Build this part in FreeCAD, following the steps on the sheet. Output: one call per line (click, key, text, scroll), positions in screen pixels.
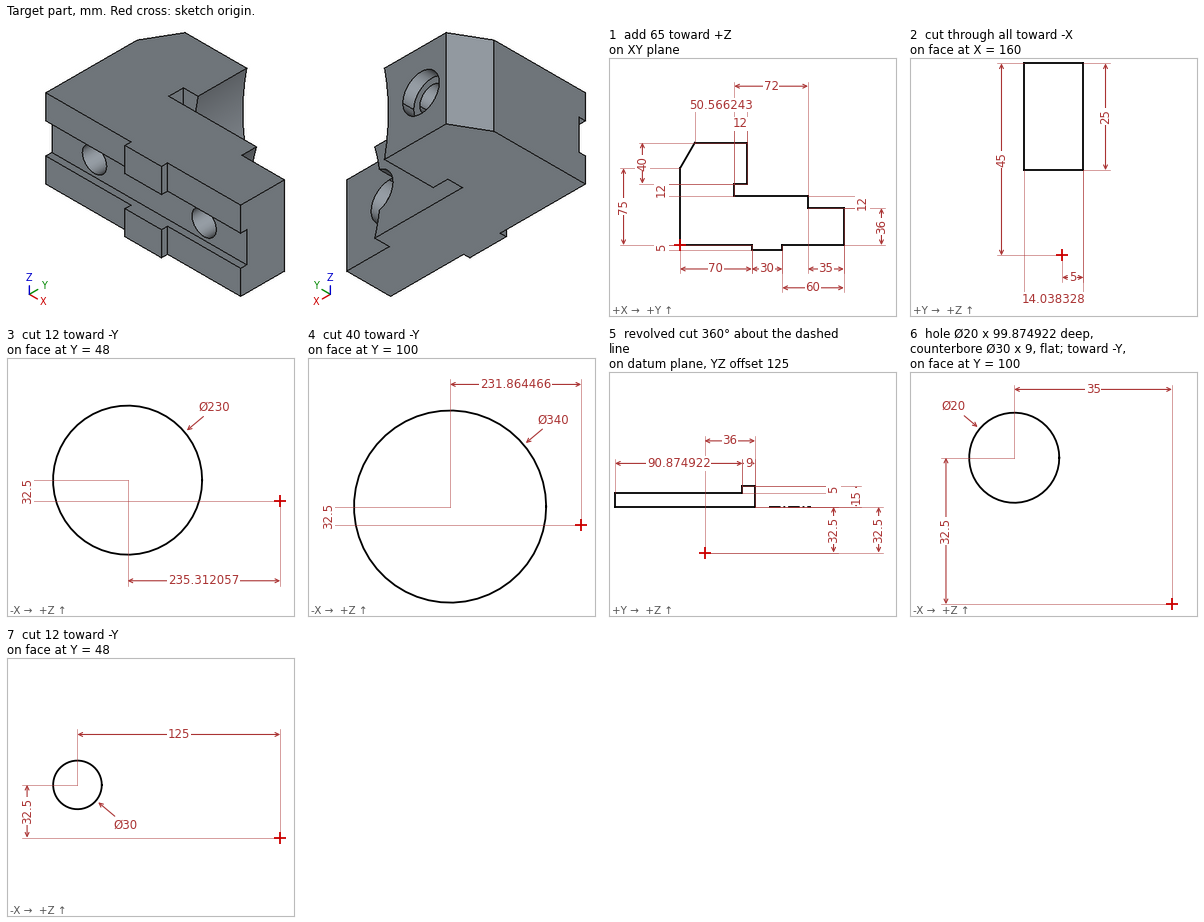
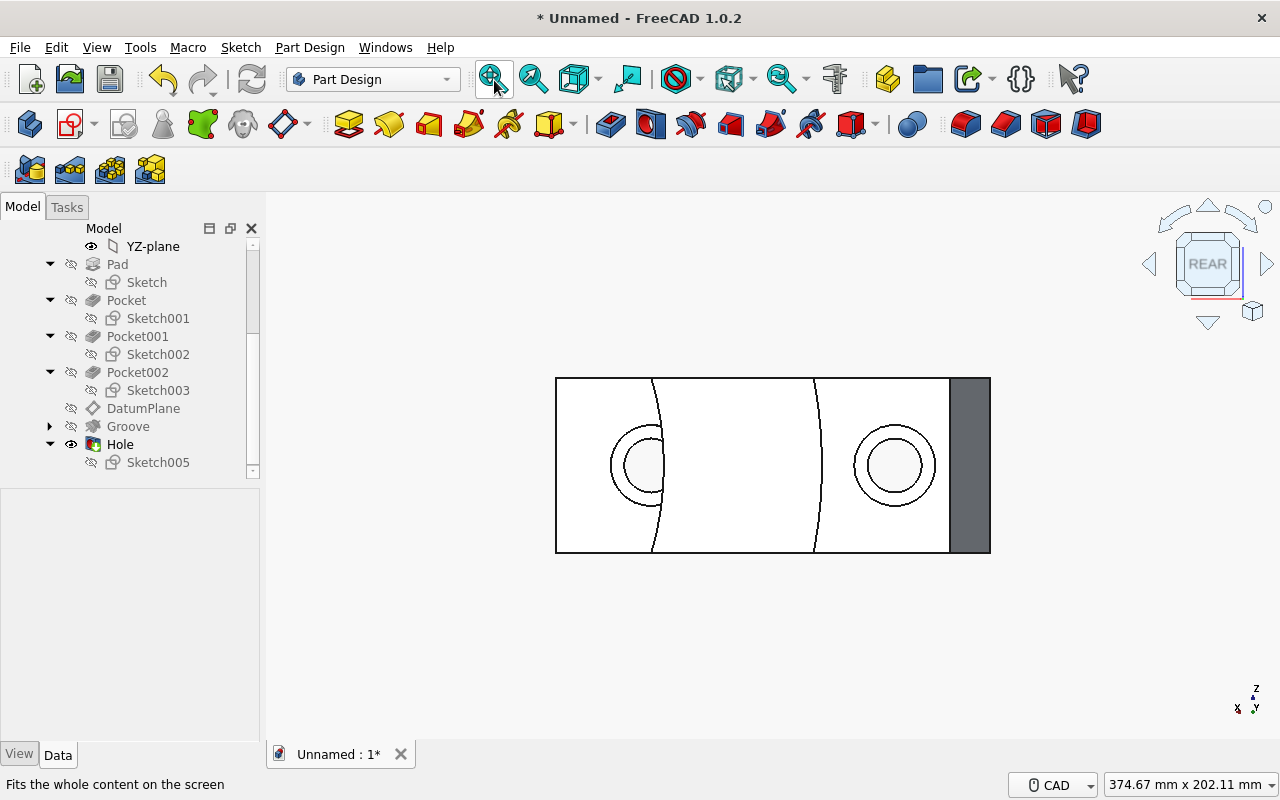
click(749, 464)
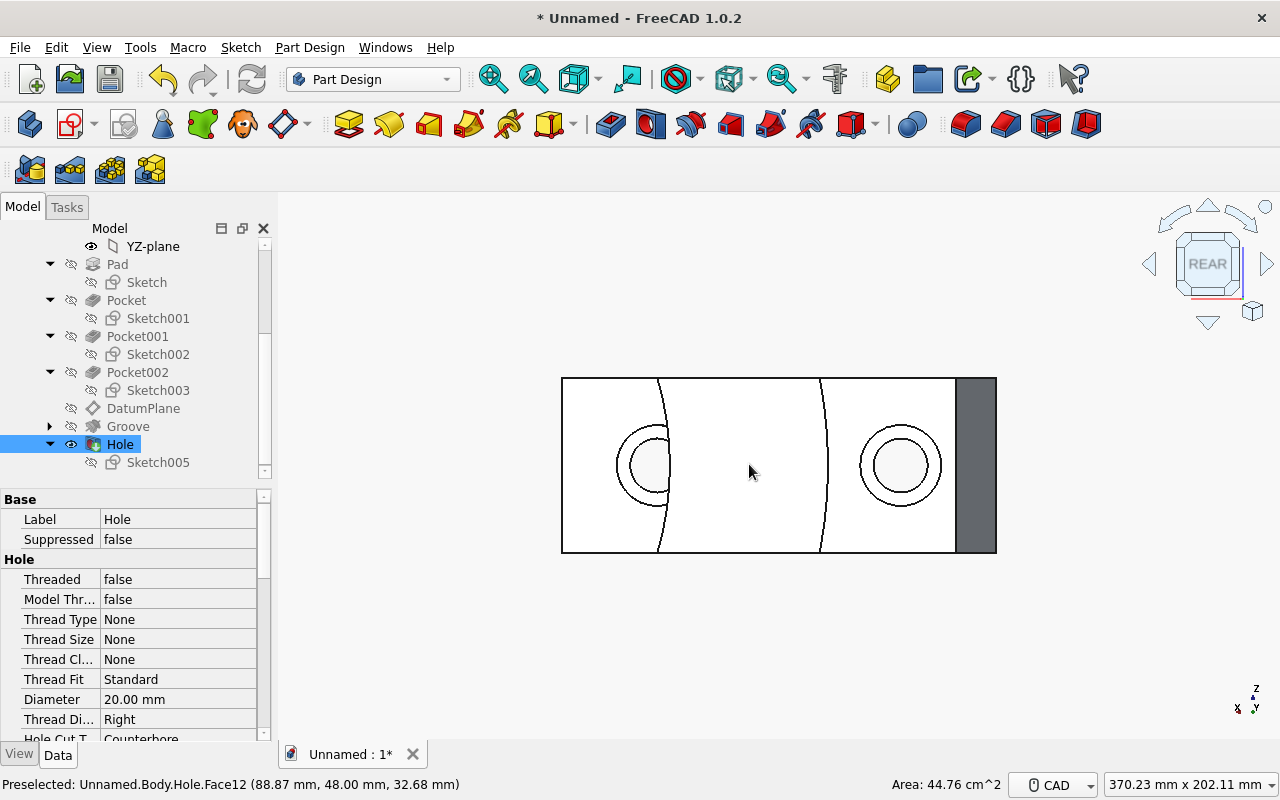
click(70, 124)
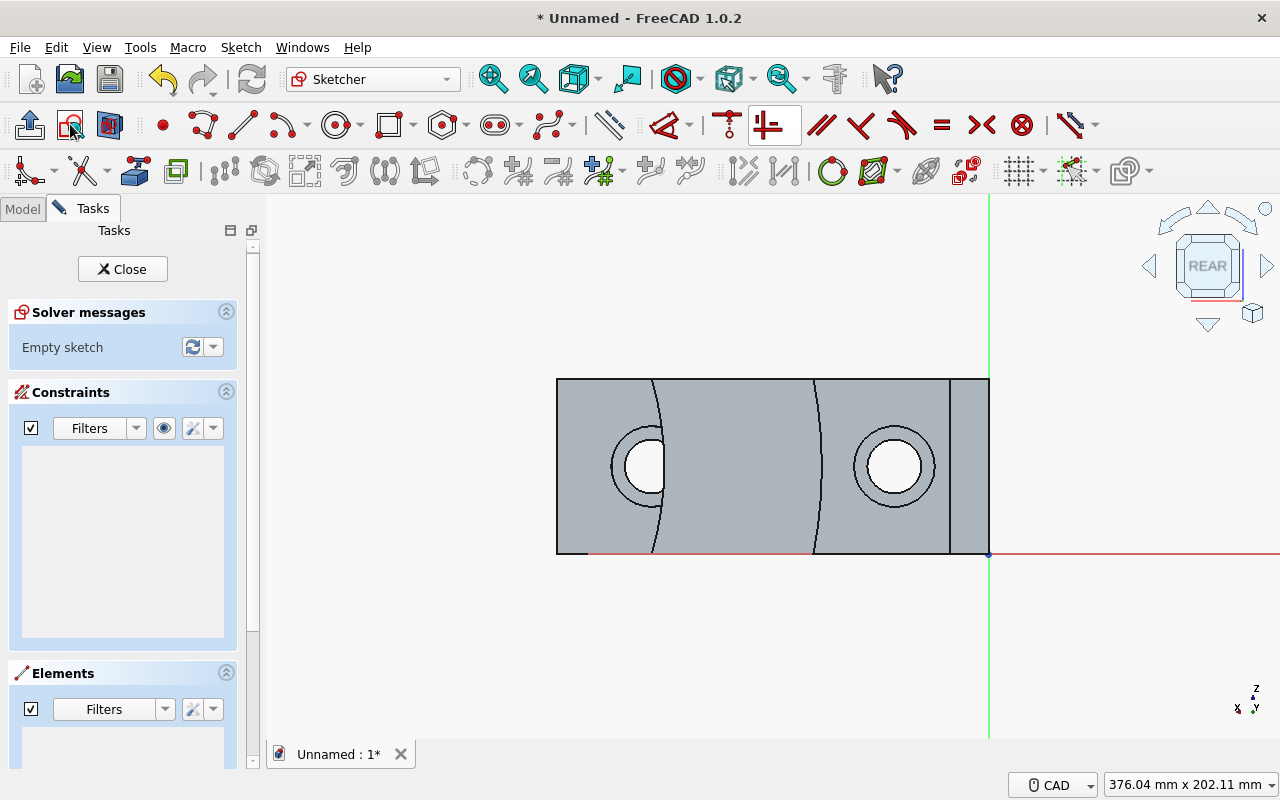
scroll(634, 466, up, 7)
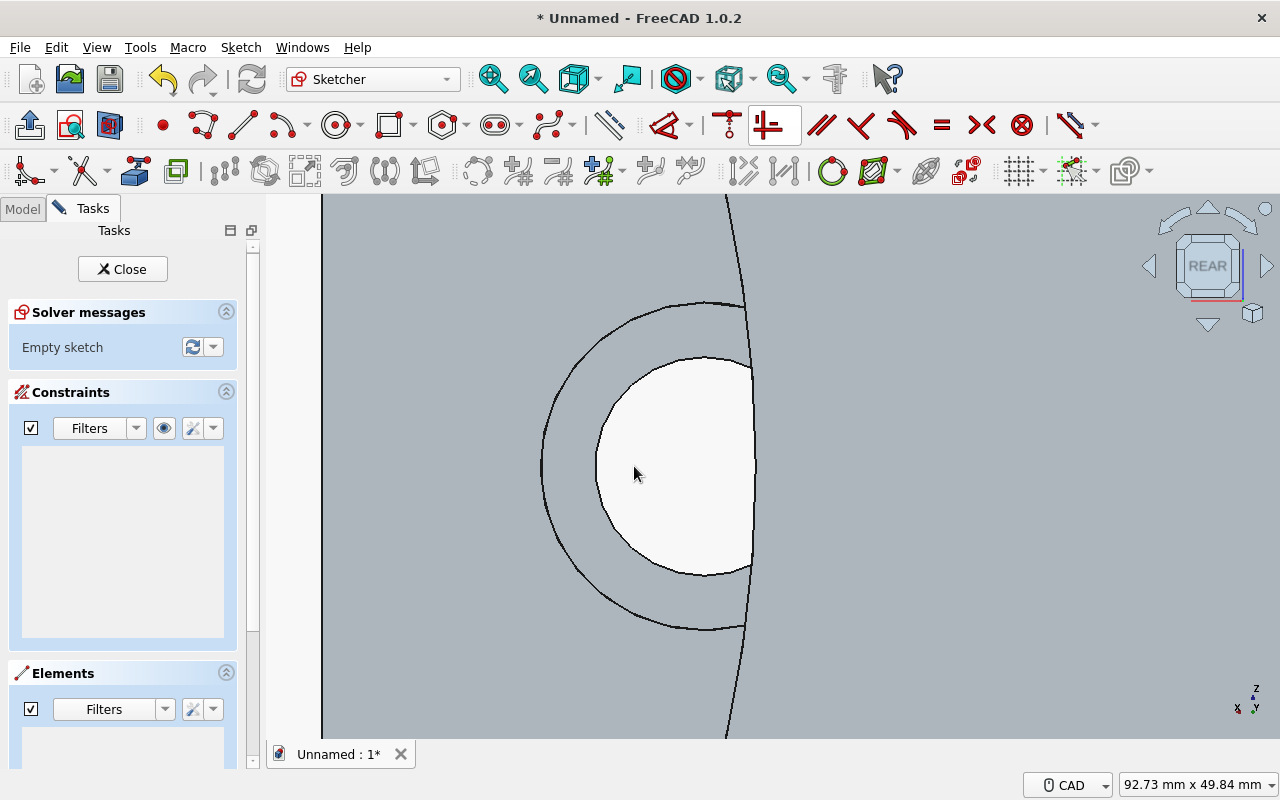
click(336, 126)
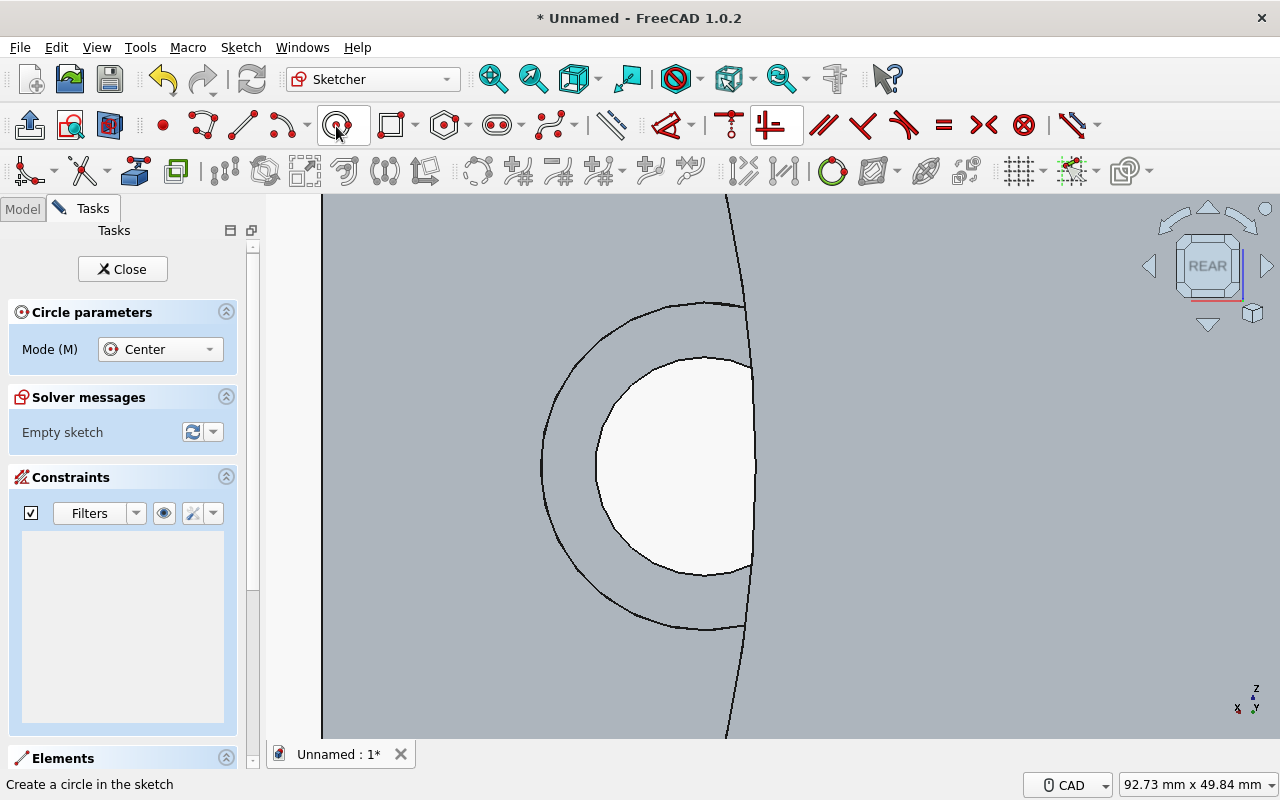
click(704, 466)
move(820, 351)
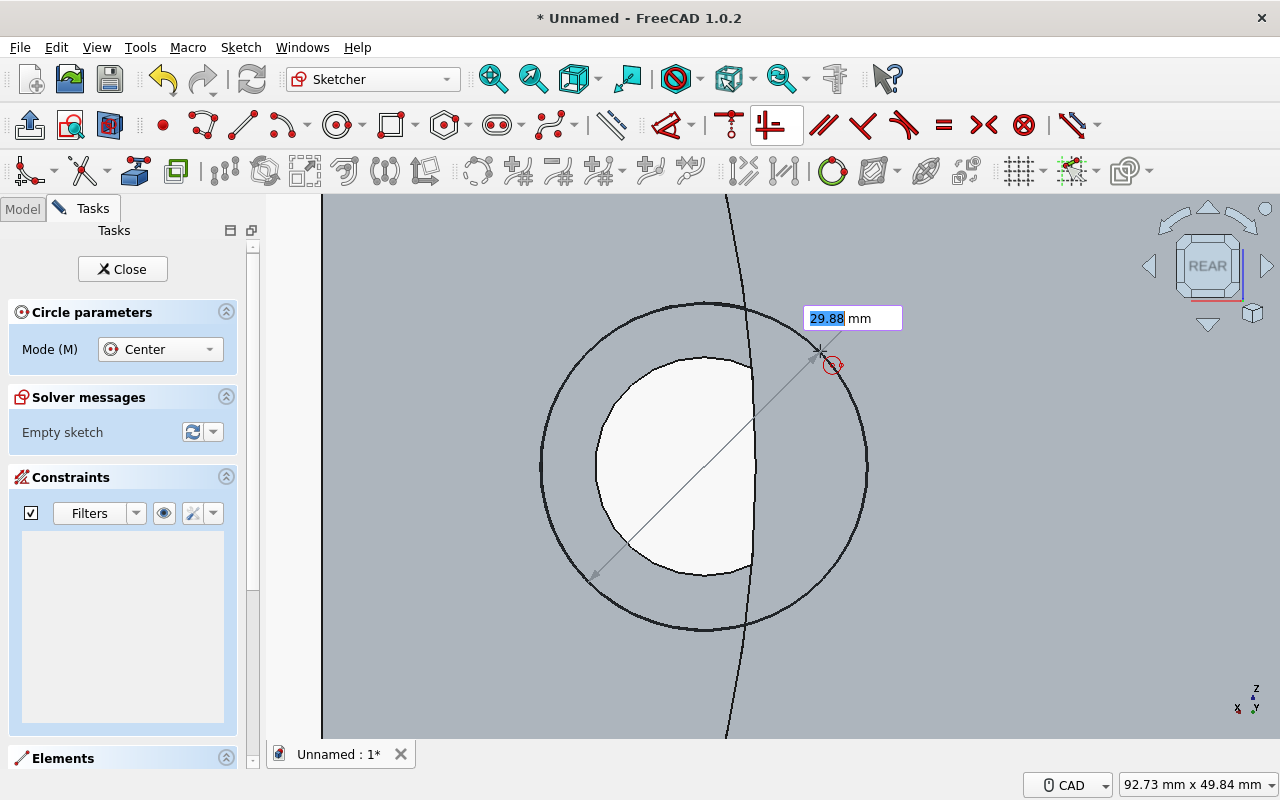
text(30)
key(Return)
key(Escape)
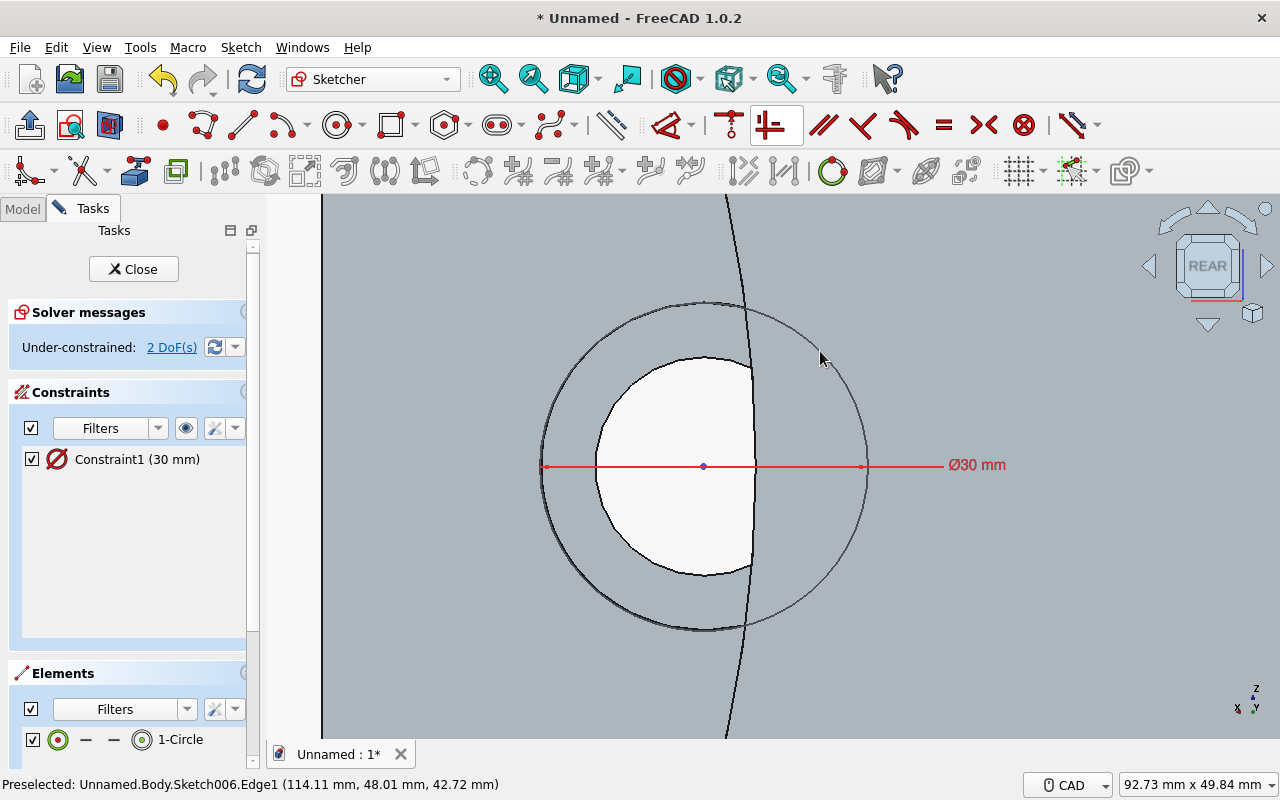
click(666, 126)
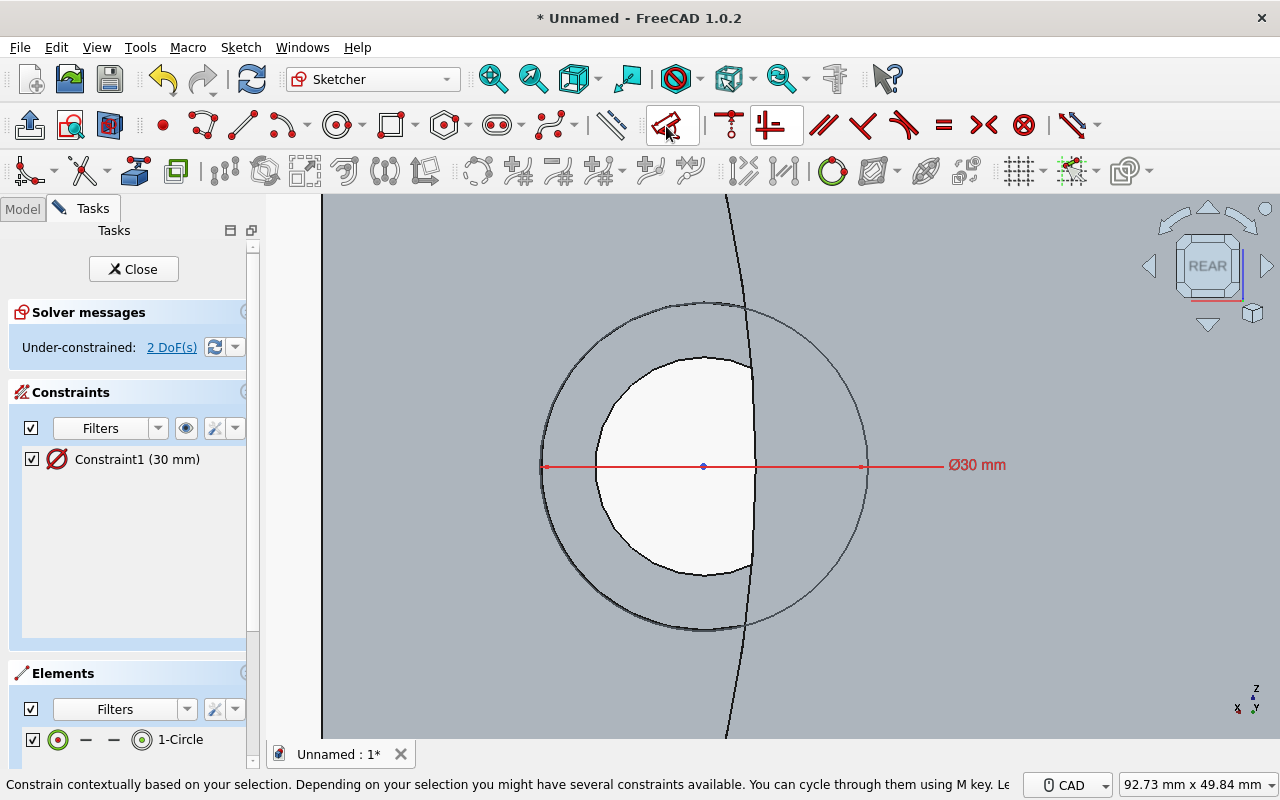
click(704, 467)
click(909, 433)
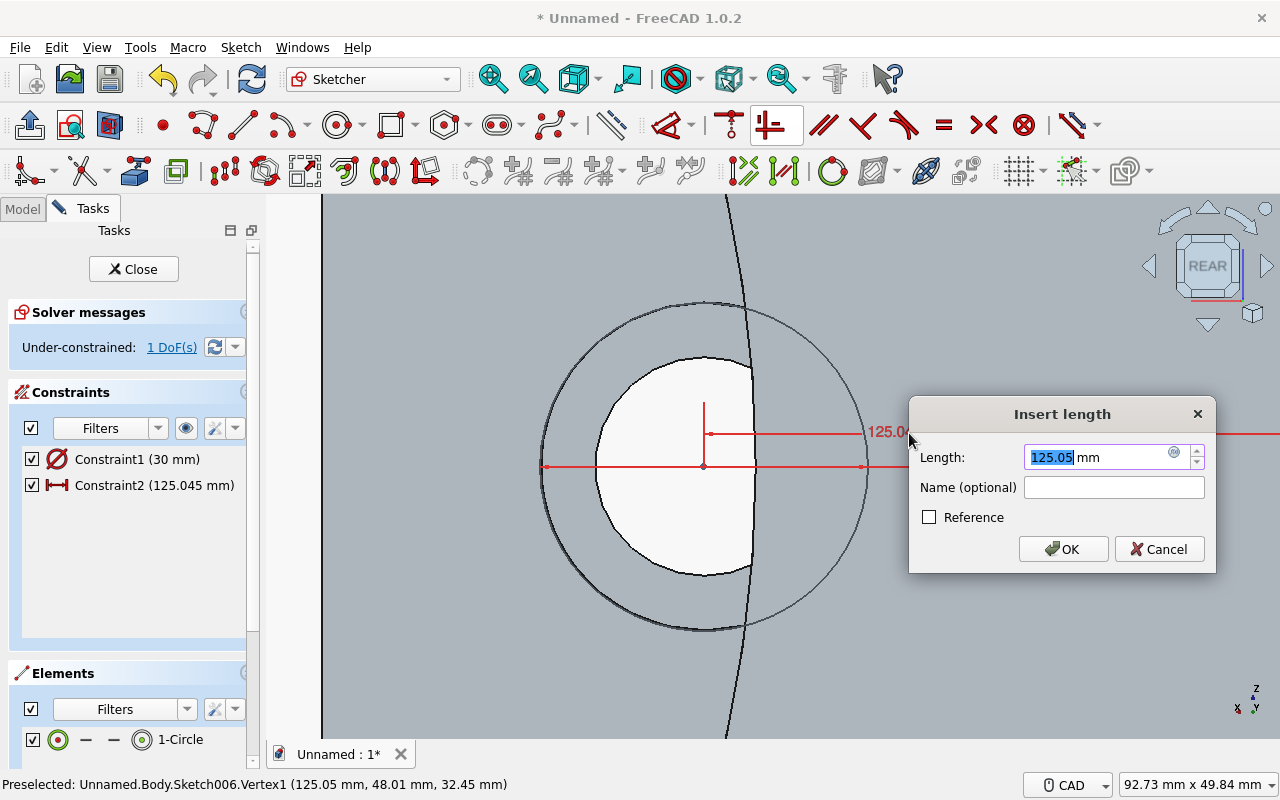
text(125)
key(Return)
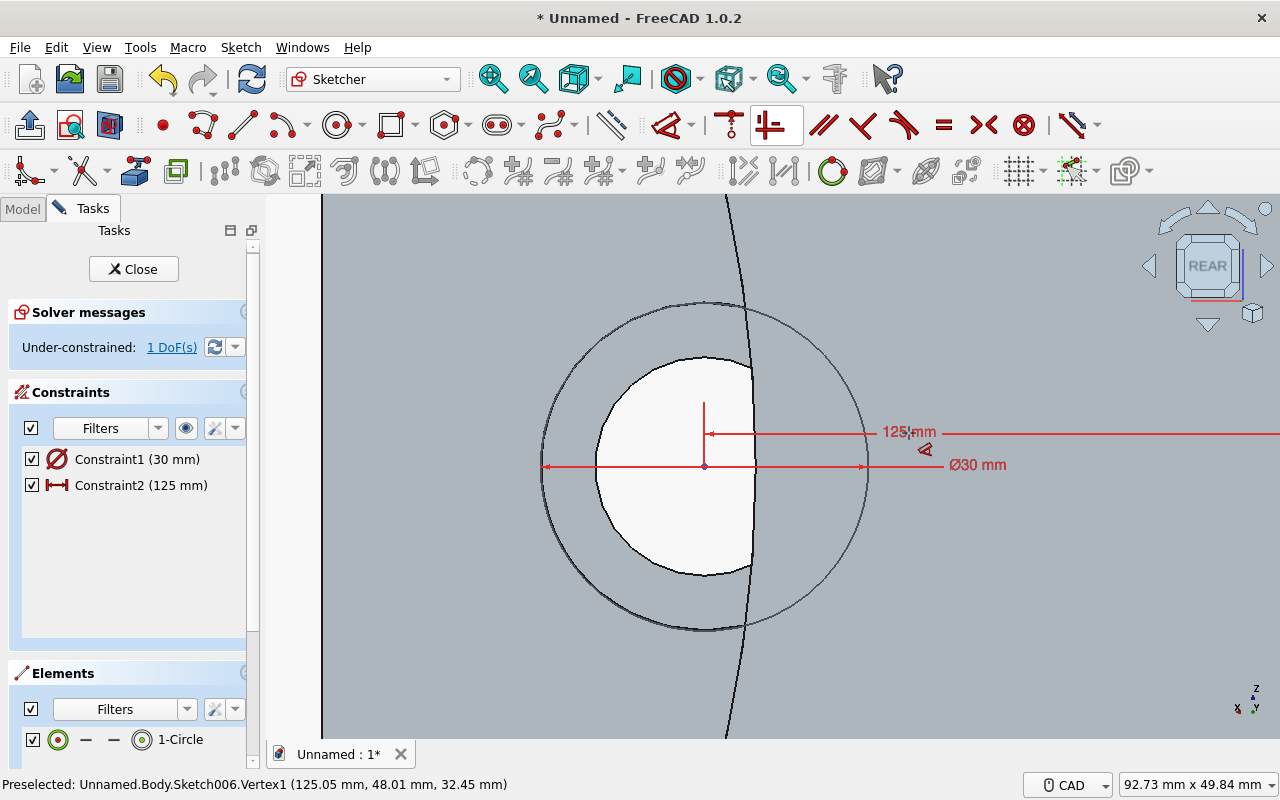
click(704, 467)
click(670, 589)